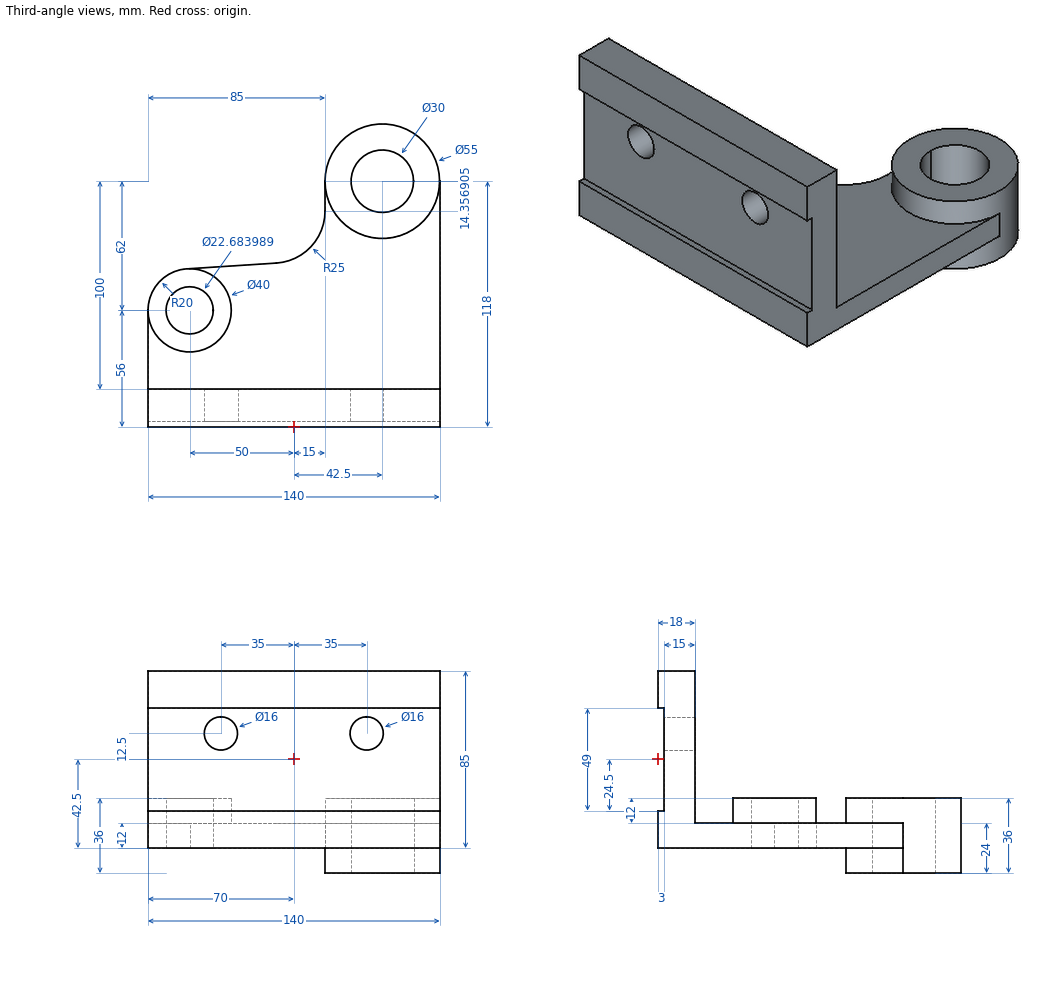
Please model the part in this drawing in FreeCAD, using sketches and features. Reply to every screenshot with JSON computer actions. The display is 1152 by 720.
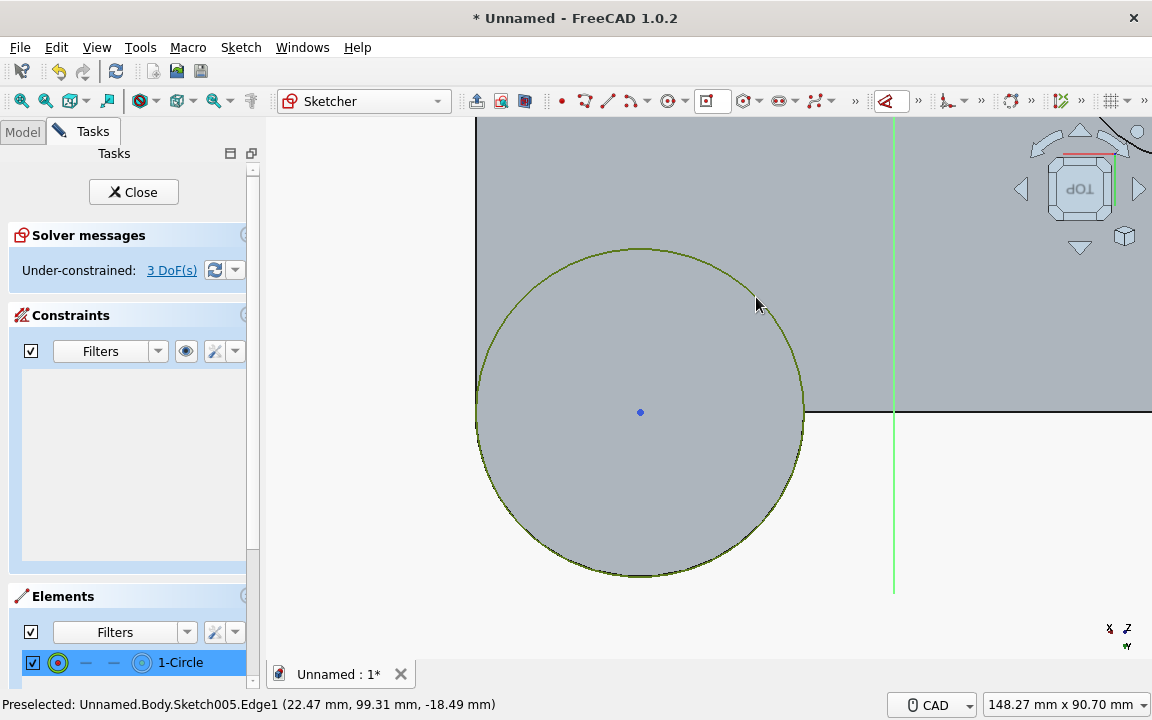
{"action": "key", "text": "k o"}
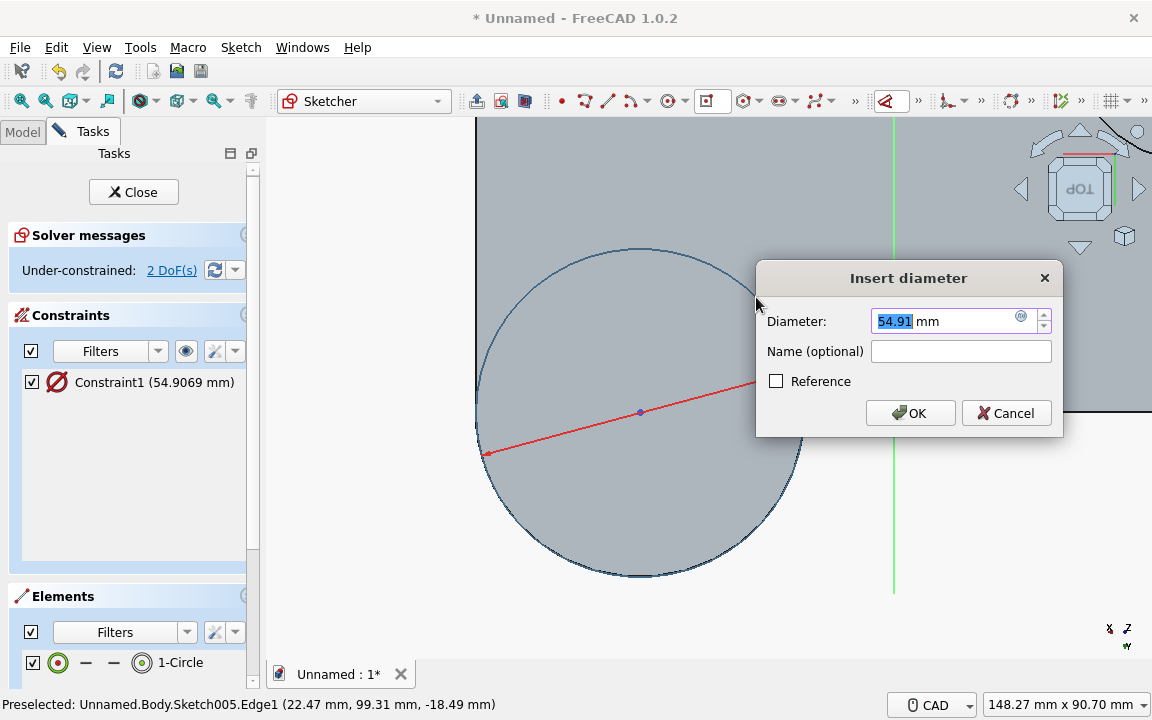
{"action": "type", "text": "55"}
{"action": "key", "text": "Return"}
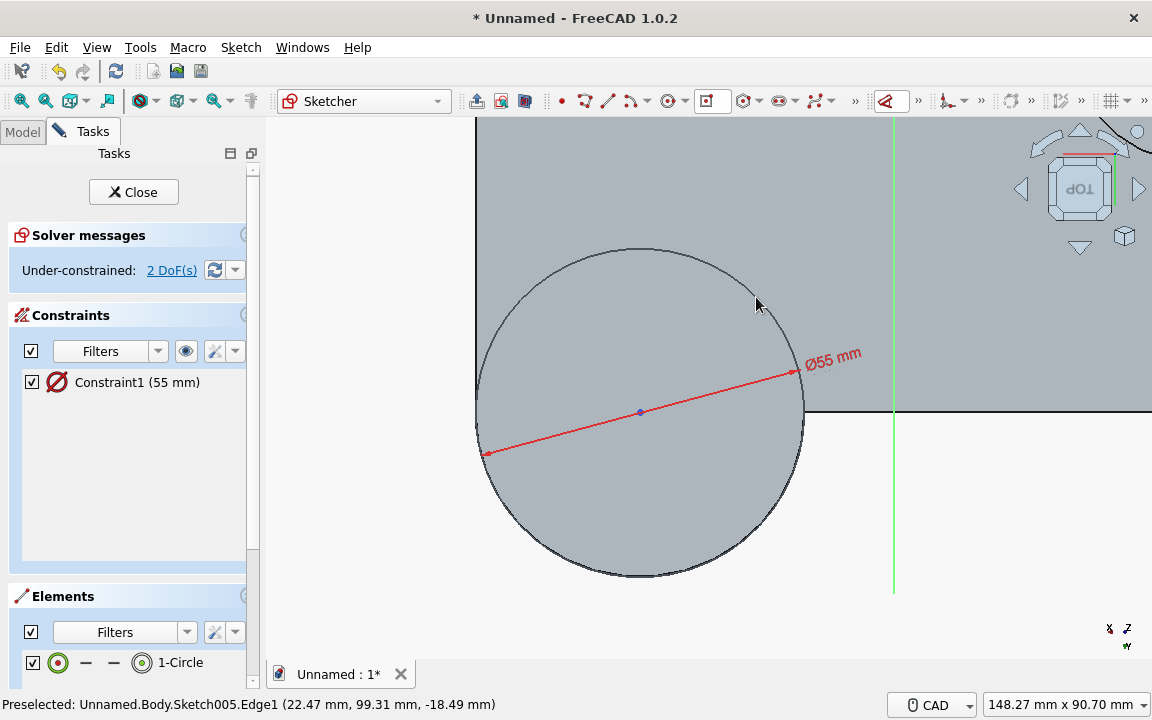
{"action": "left_click", "coordinate": [640, 413]}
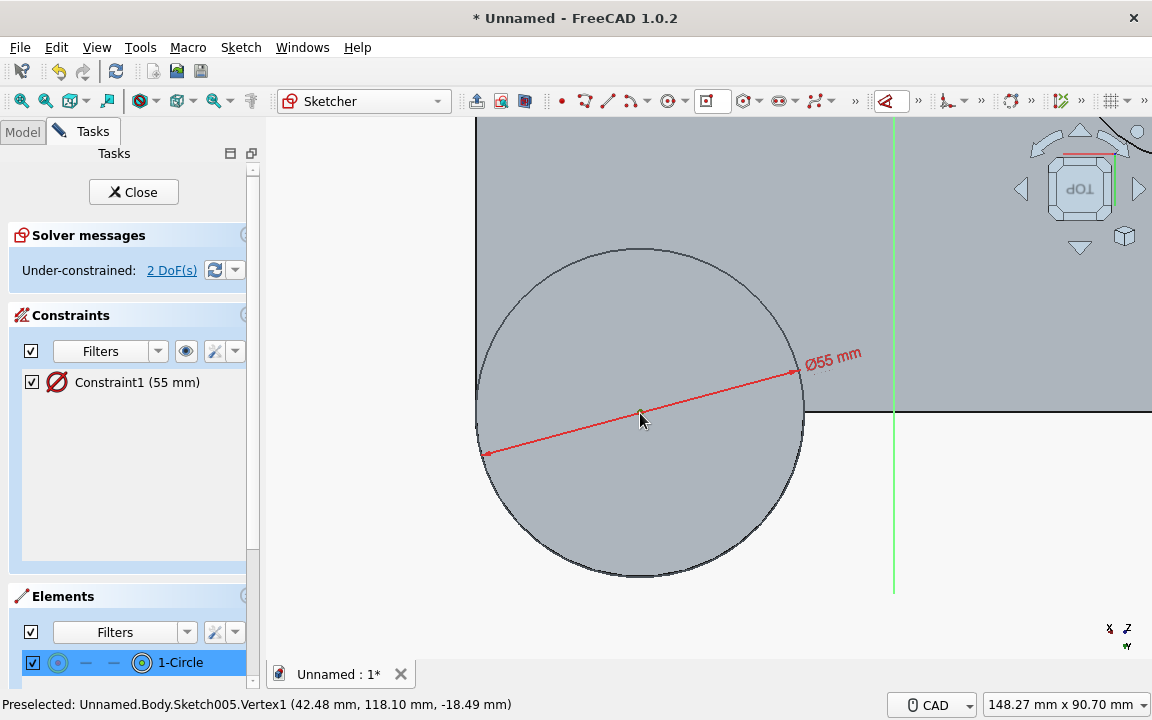
{"action": "left_click", "coordinate": [904, 102]}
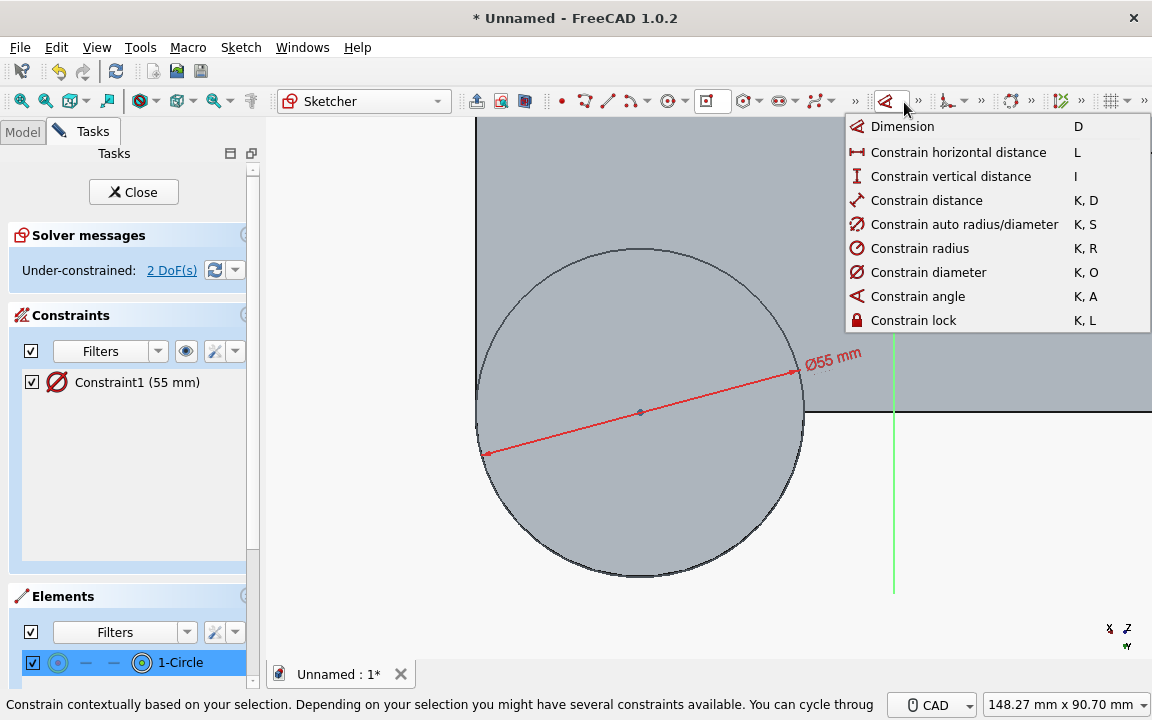
{"action": "left_click", "coordinate": [998, 176]}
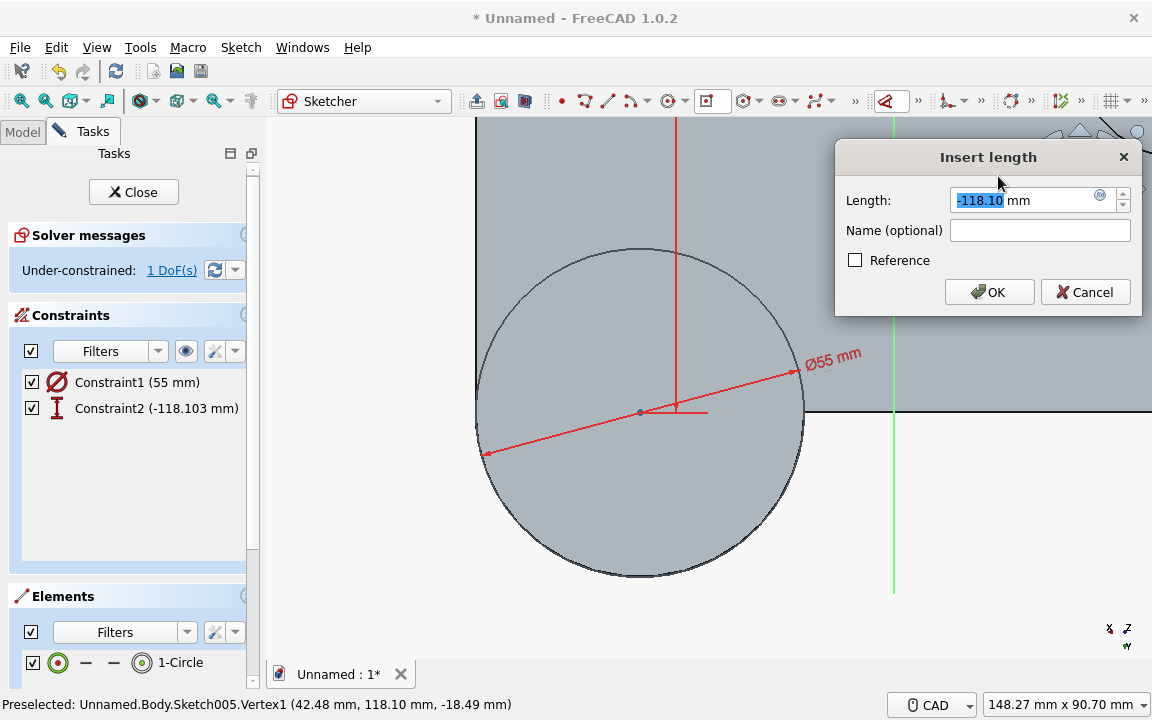
{"action": "type", "text": "-118"}
{"action": "key", "text": "Return"}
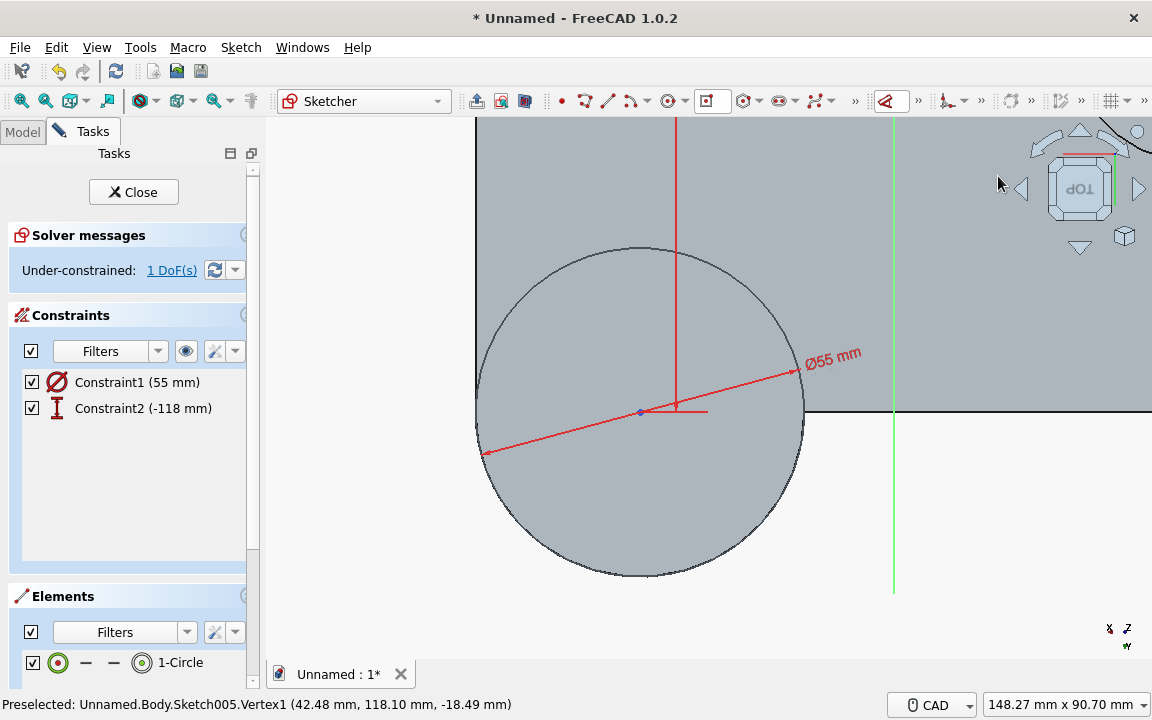
{"action": "left_click", "coordinate": [640, 412]}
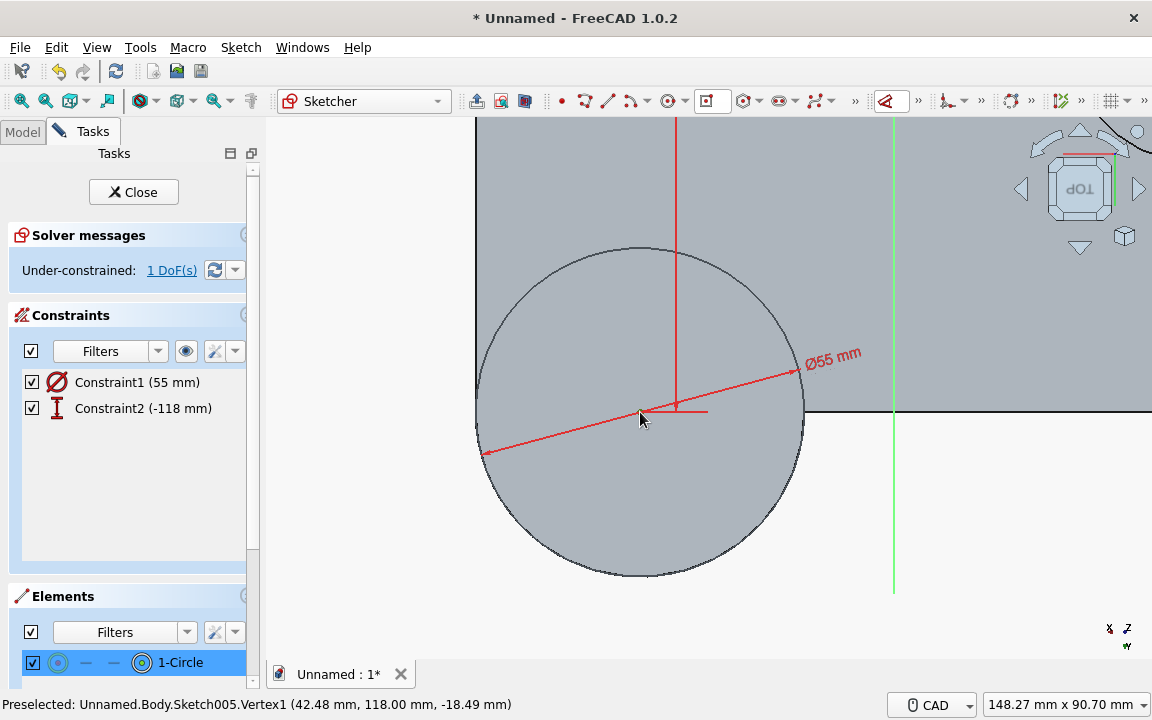
{"action": "key", "text": "l"}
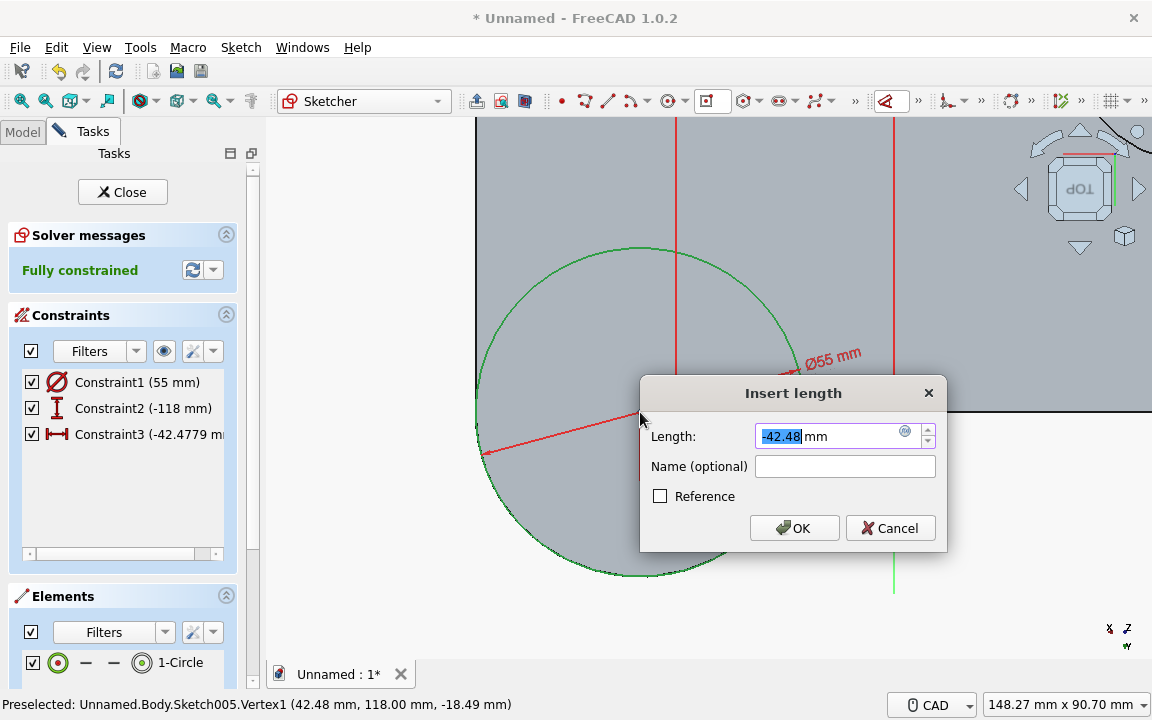
{"action": "type", "text": "-42.5"}
{"action": "key", "text": "Return"}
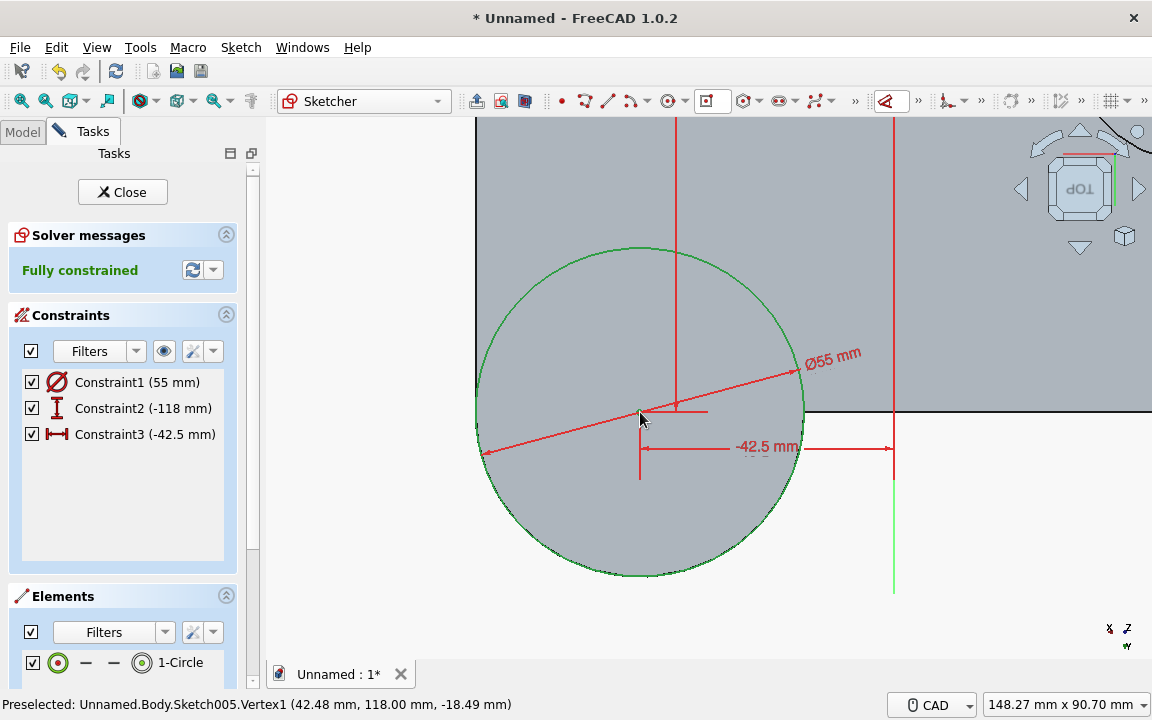
{"action": "left_click", "coordinate": [123, 192]}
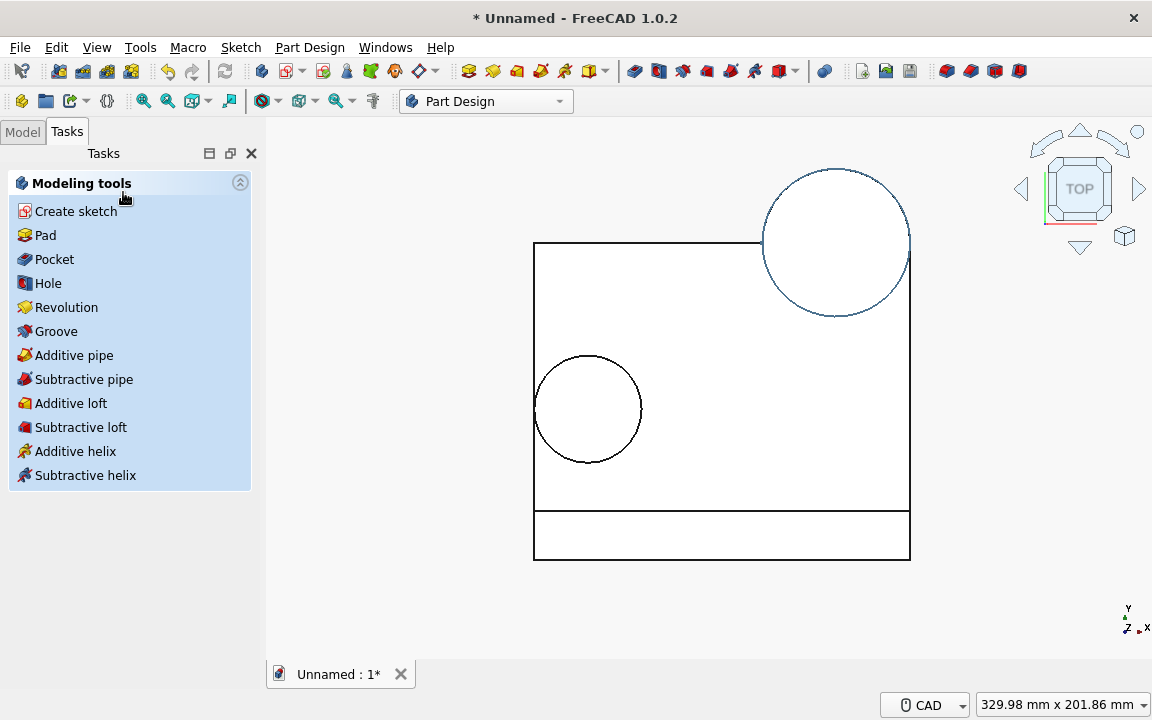
{"action": "left_click", "coordinate": [470, 72]}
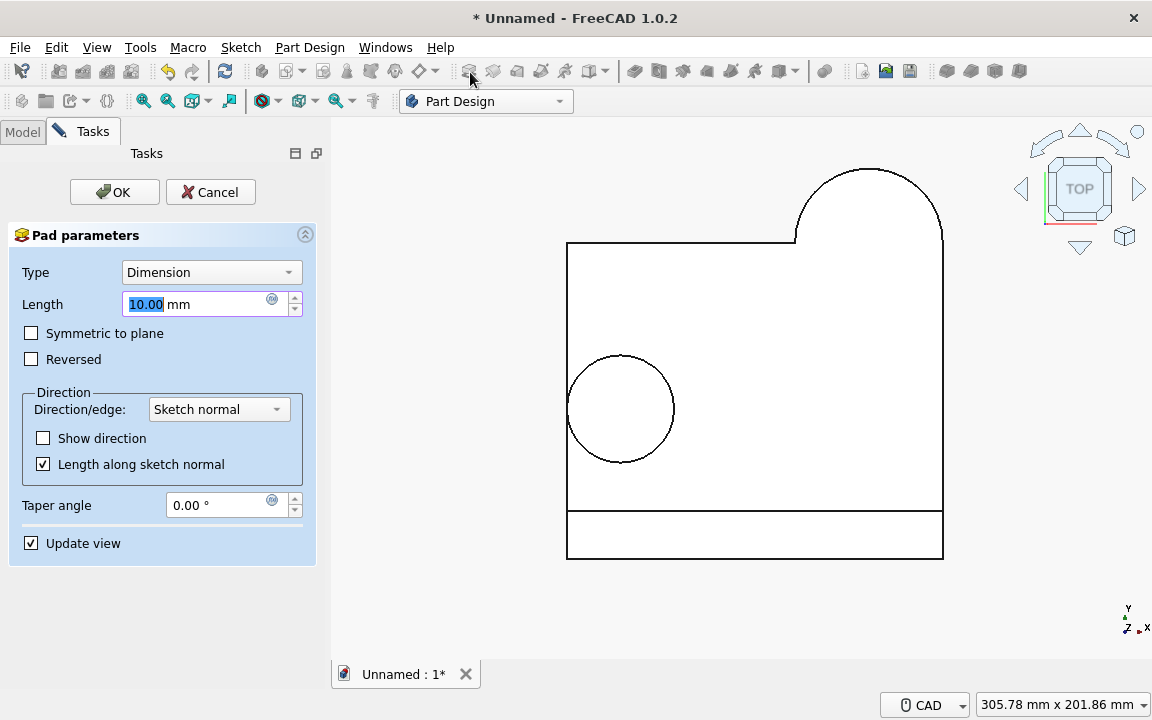
{"action": "type", "text": "12"}
{"action": "key", "text": "Tab"}